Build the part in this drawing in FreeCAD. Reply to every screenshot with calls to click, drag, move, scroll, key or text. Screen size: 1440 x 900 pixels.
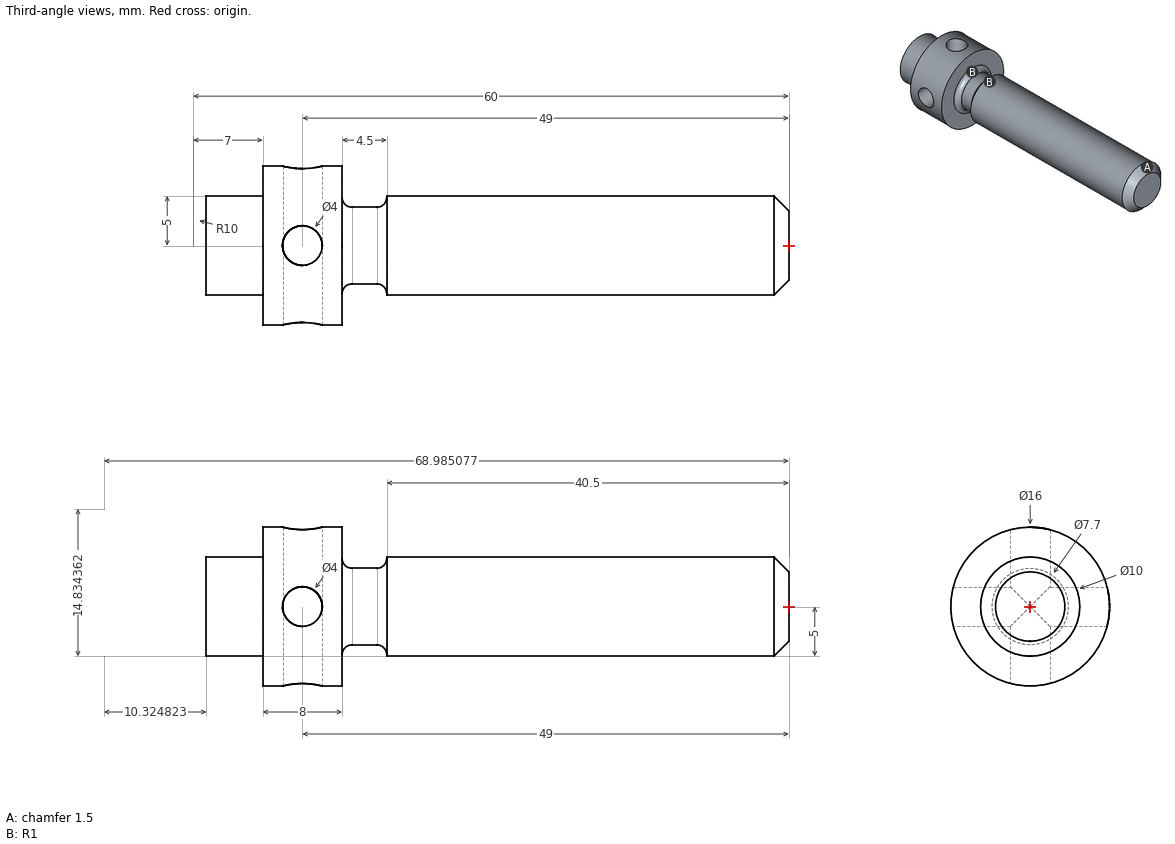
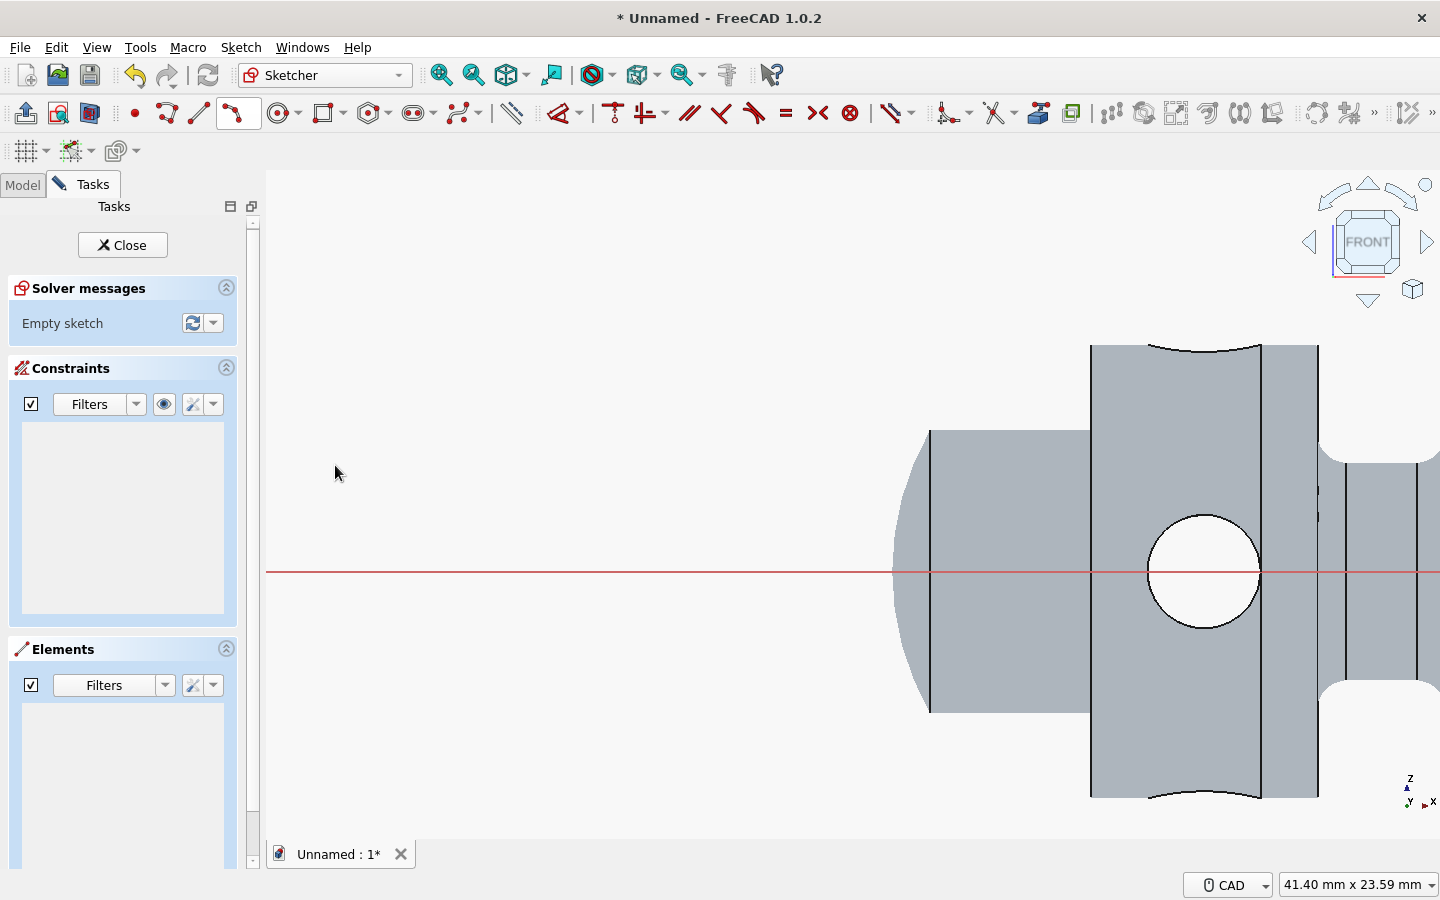
key(g)
key(r)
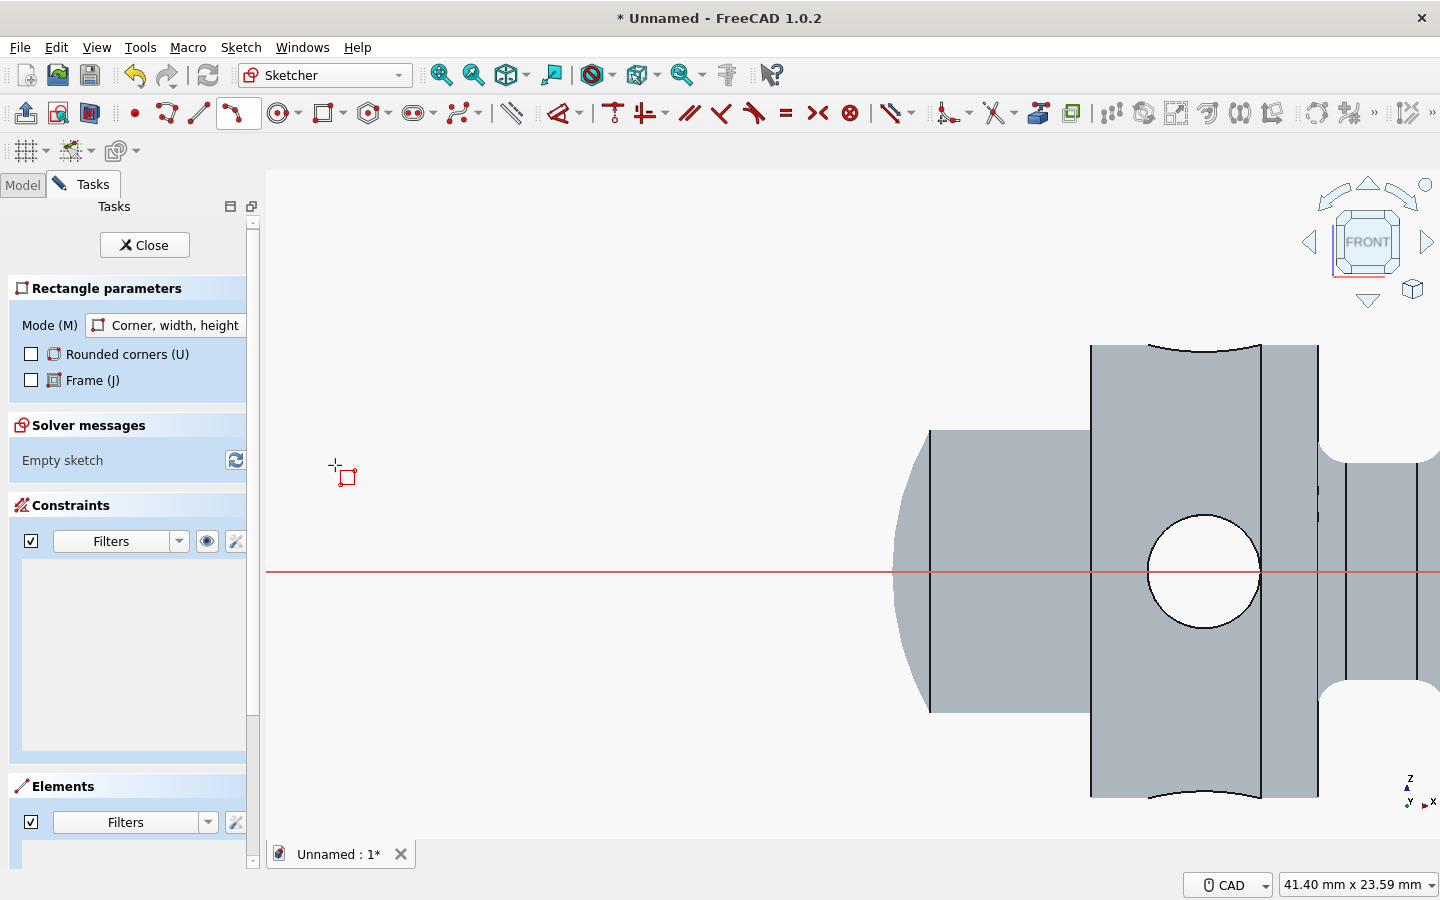
click(637, 293)
click(930, 713)
key(Escape)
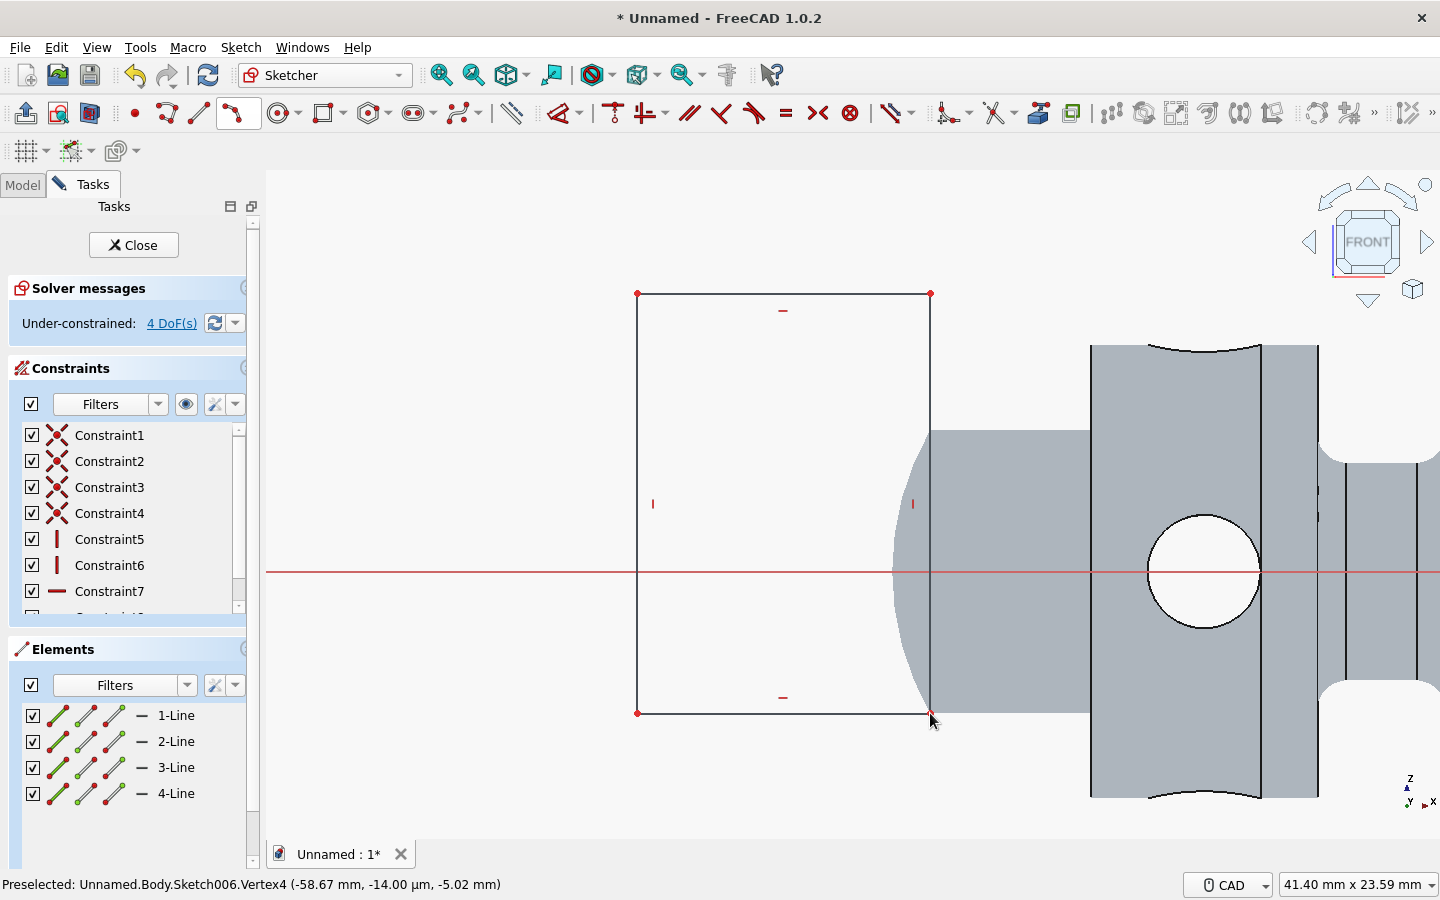
key(d)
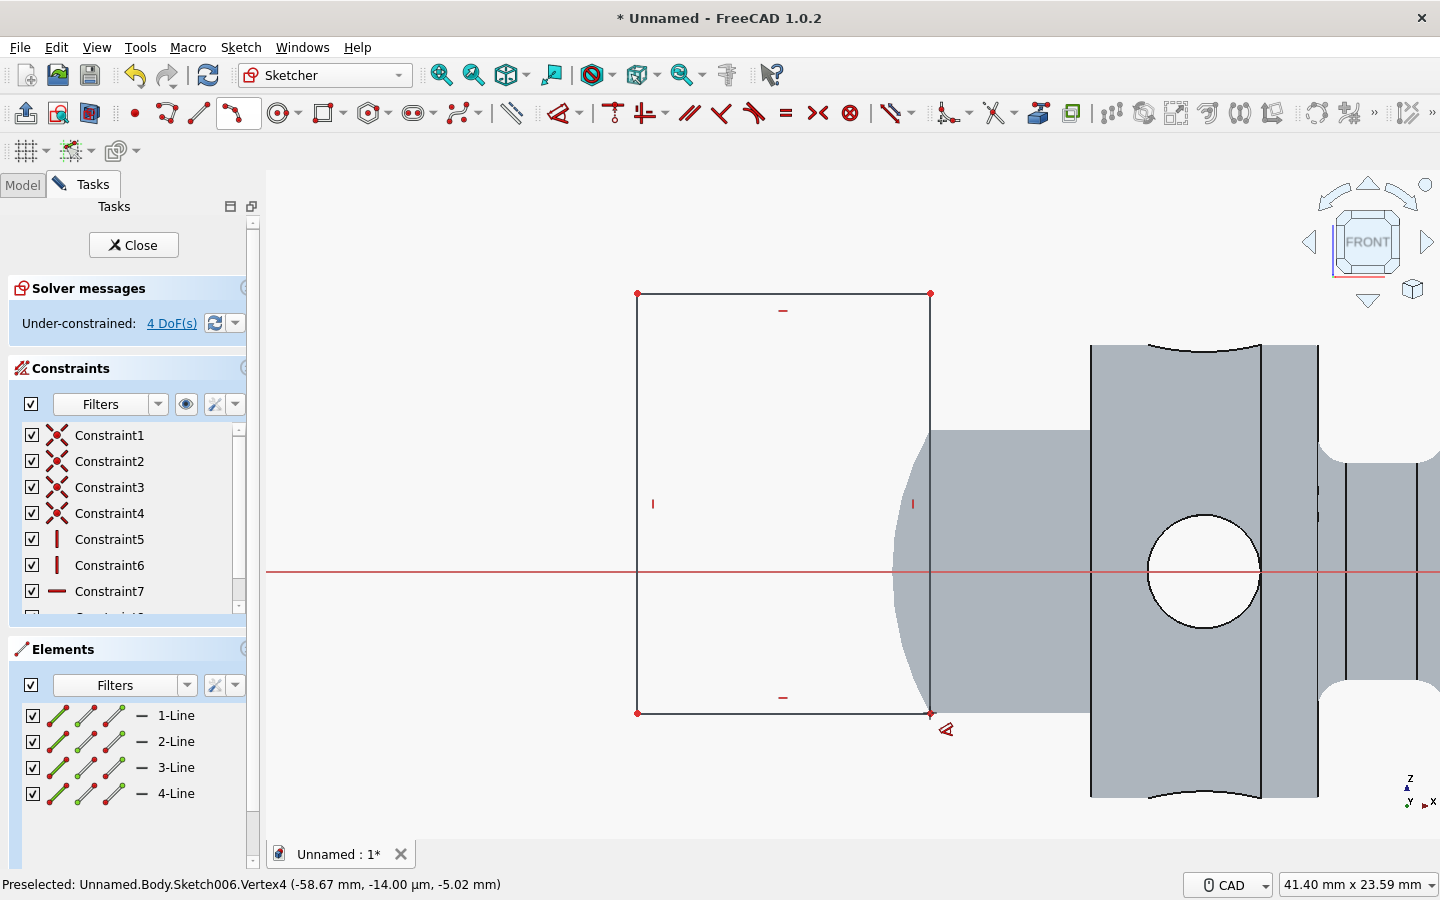
click(637, 714)
click(603, 643)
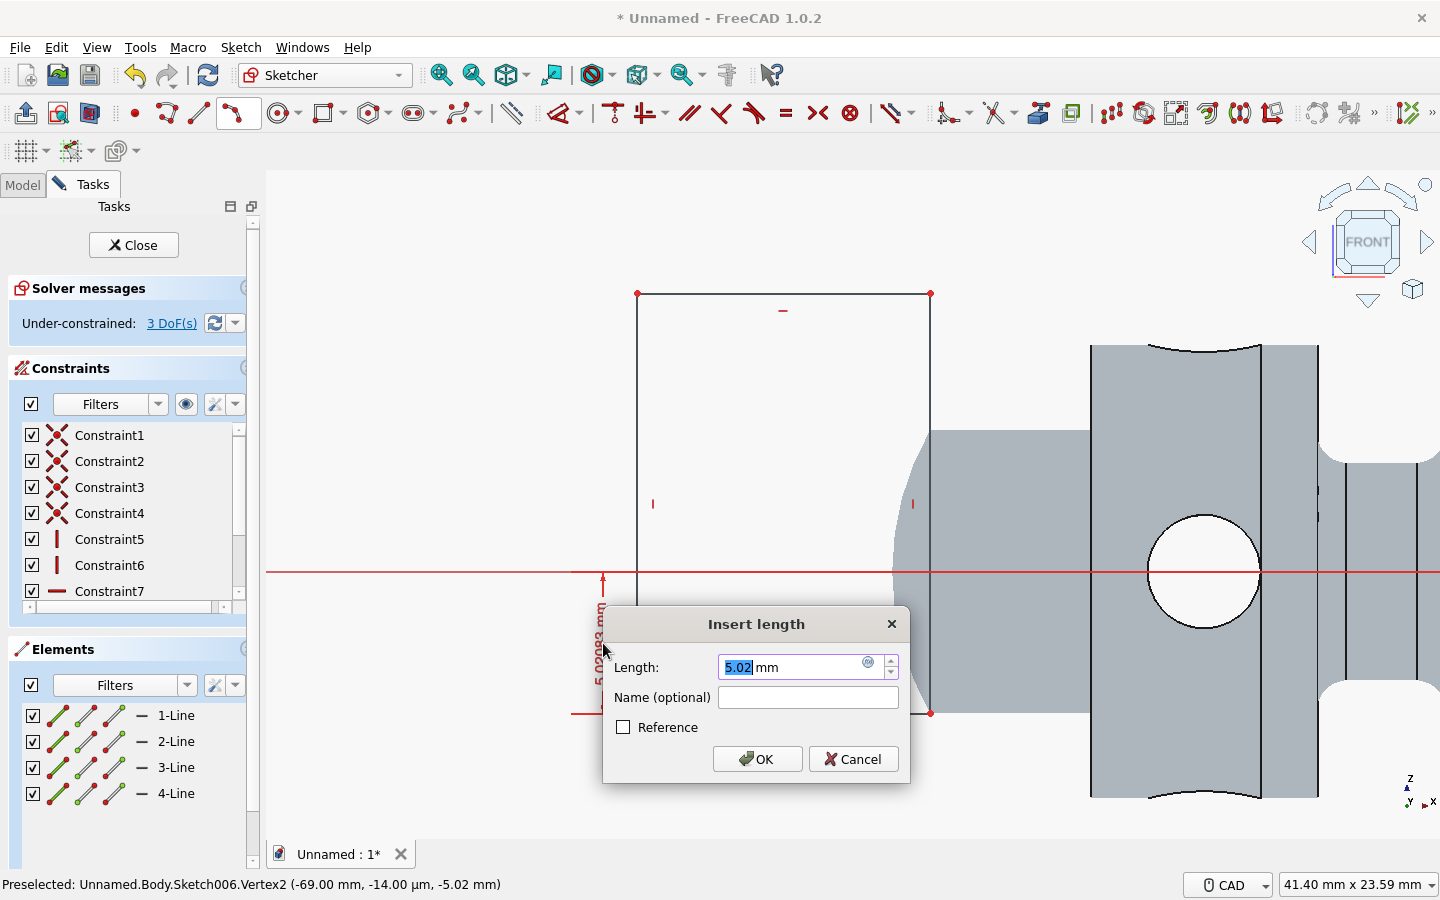
text(5)
key(Return)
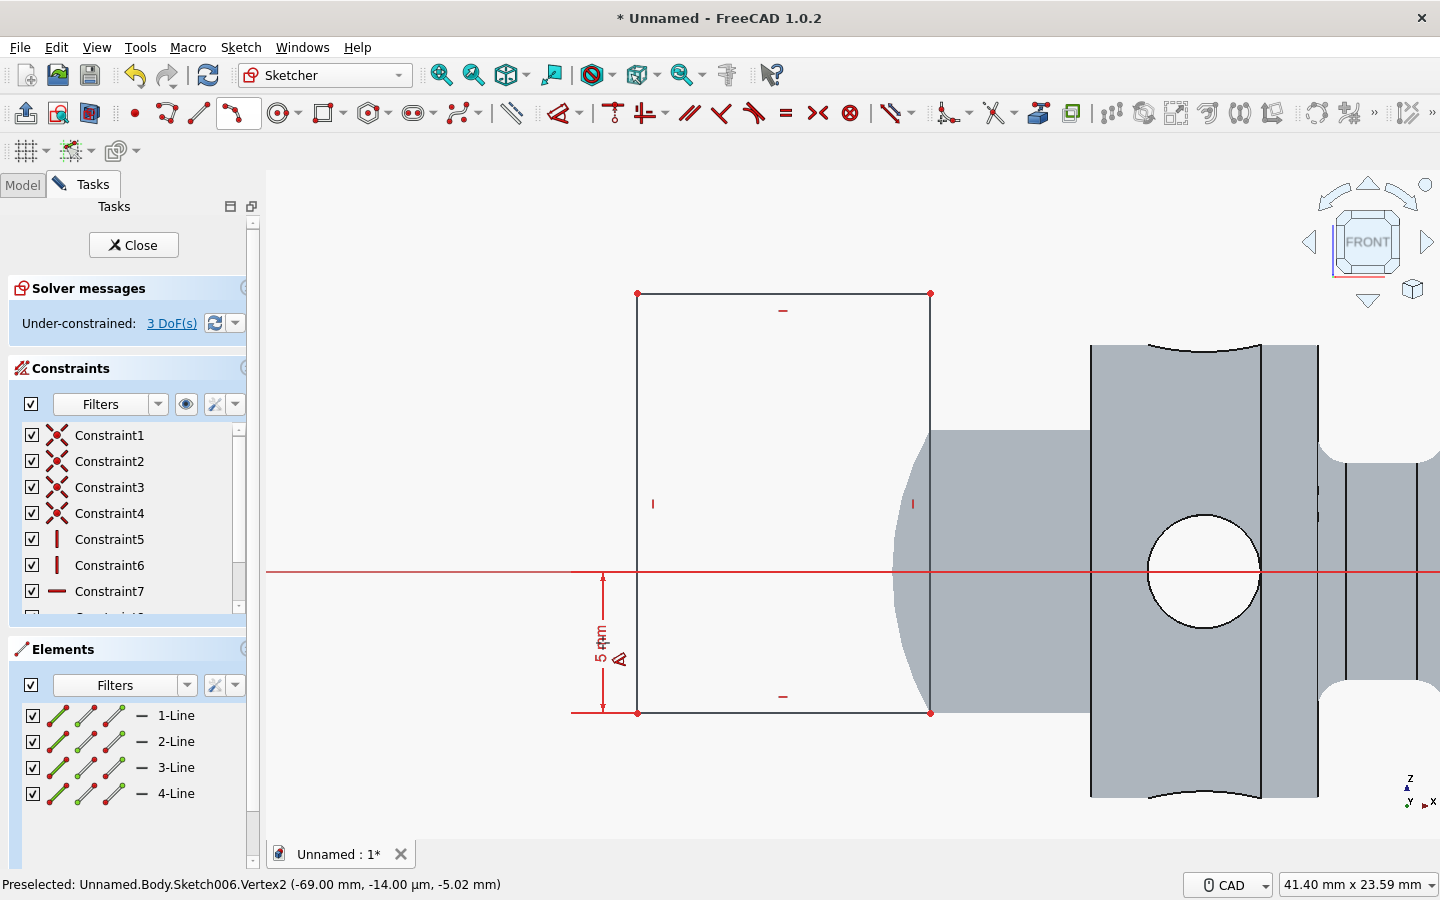
click(637, 420)
click(603, 504)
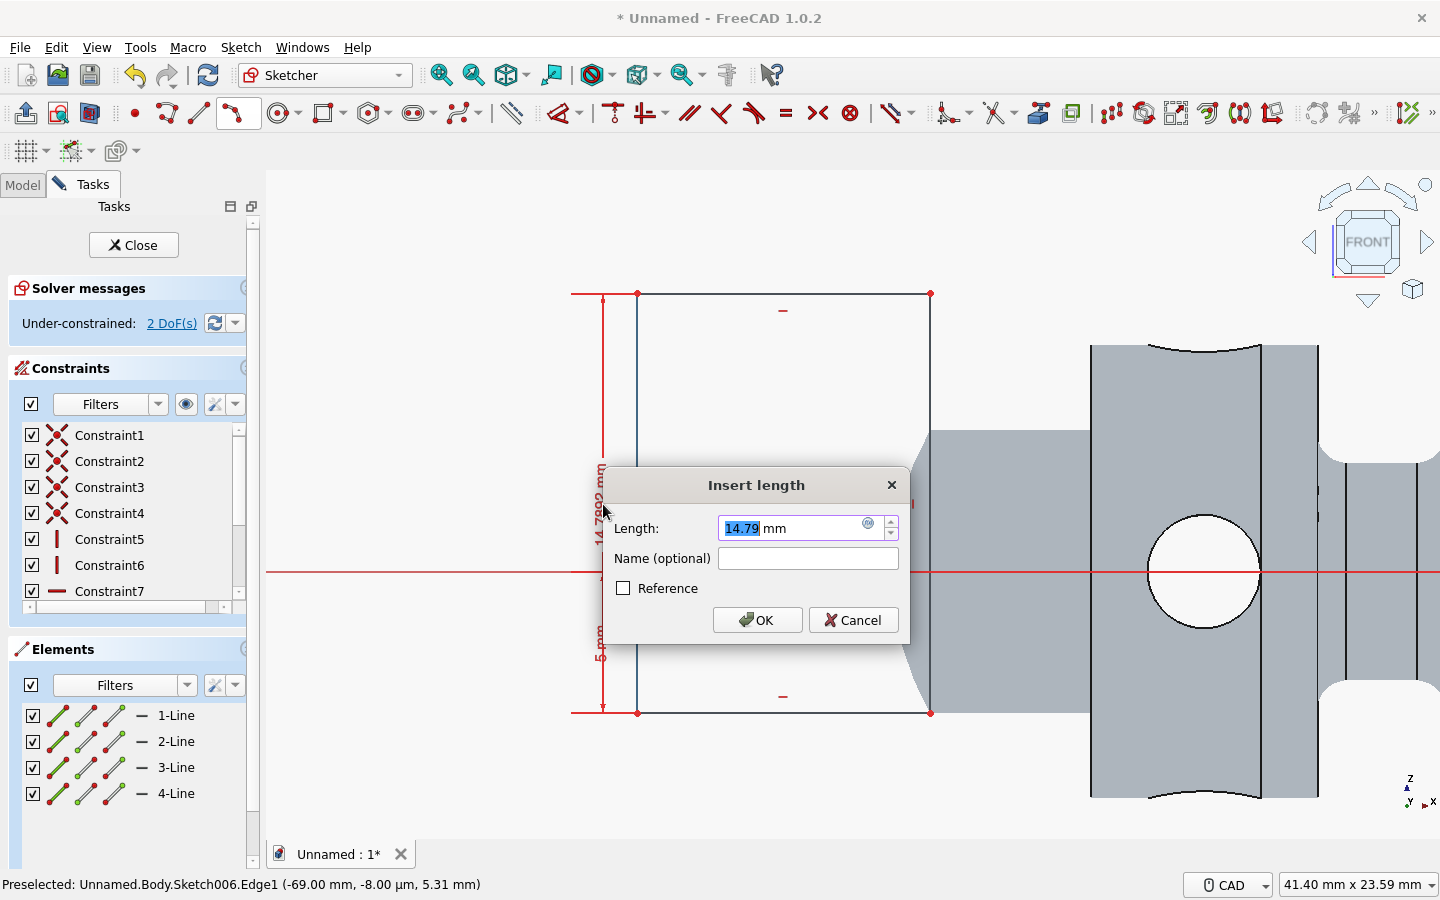
text(14.834362)
key(Return)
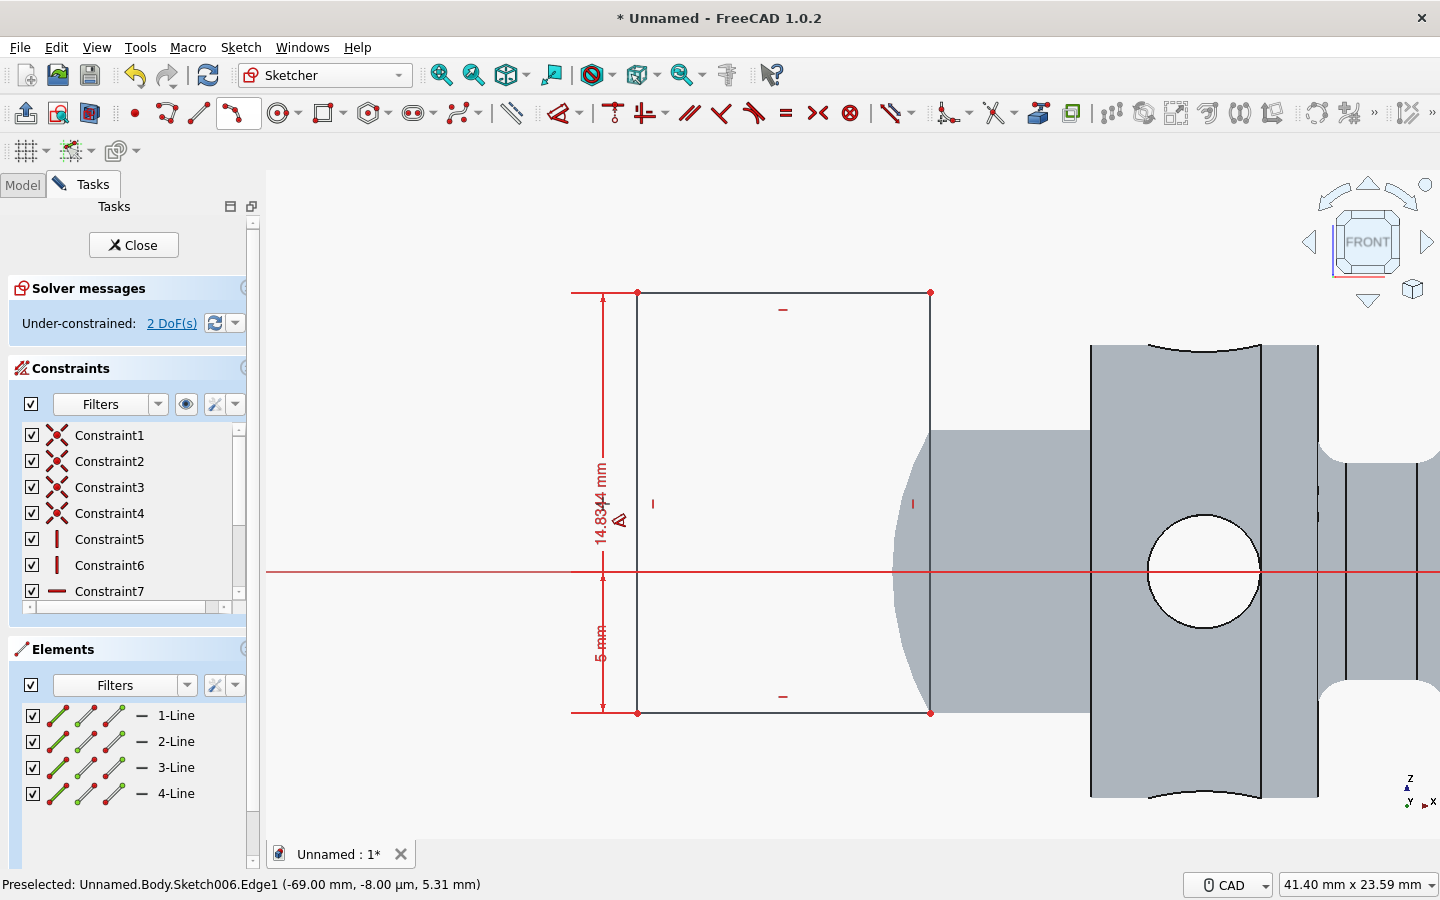
click(725, 713)
click(783, 747)